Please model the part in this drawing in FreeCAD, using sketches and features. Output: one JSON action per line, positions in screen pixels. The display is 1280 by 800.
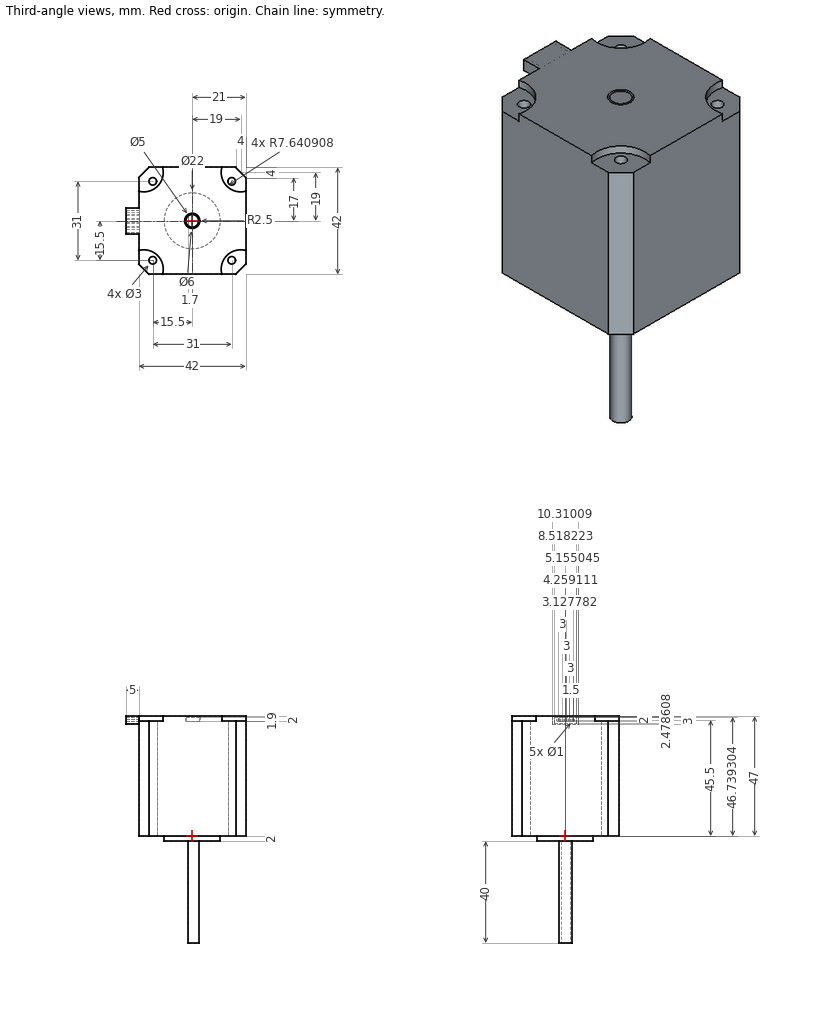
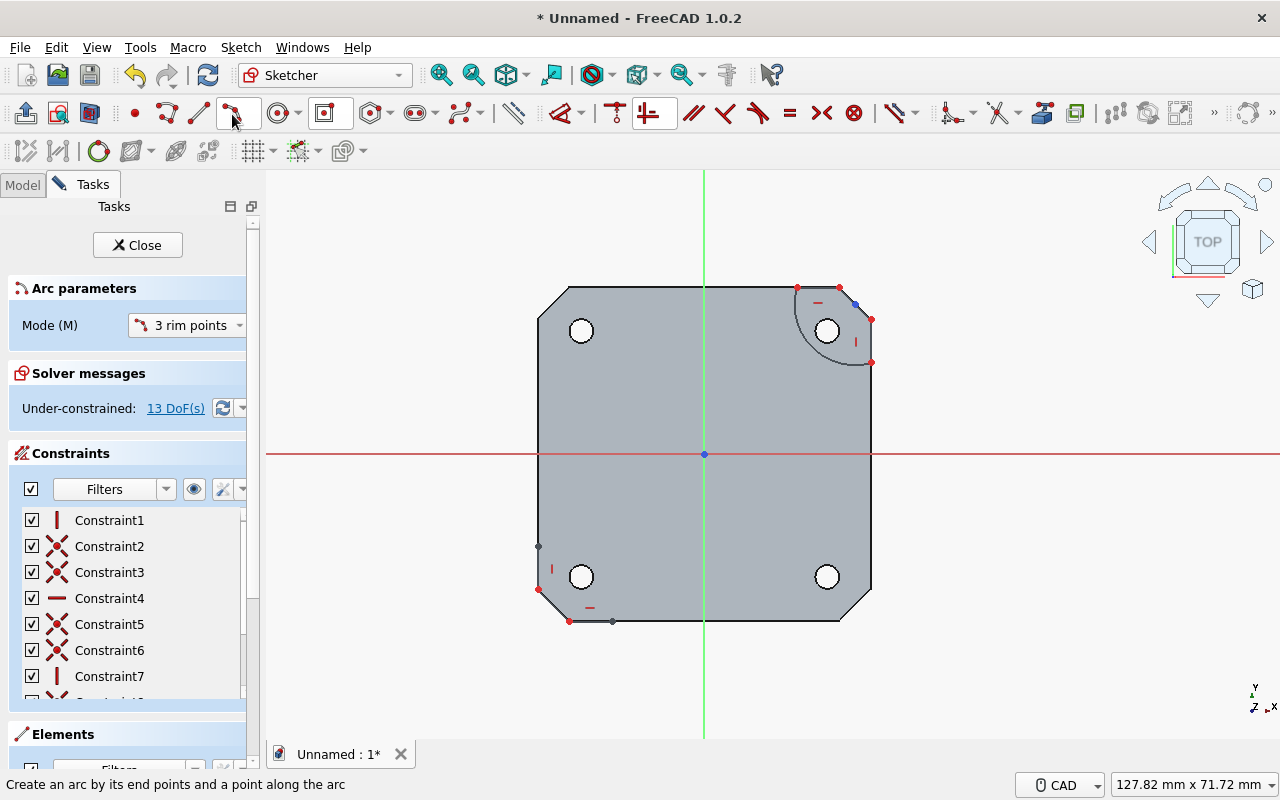
{"action": "left_click", "coordinate": [612, 622]}
{"action": "left_click", "coordinate": [538, 547]}
{"action": "left_click", "coordinate": [596, 562]}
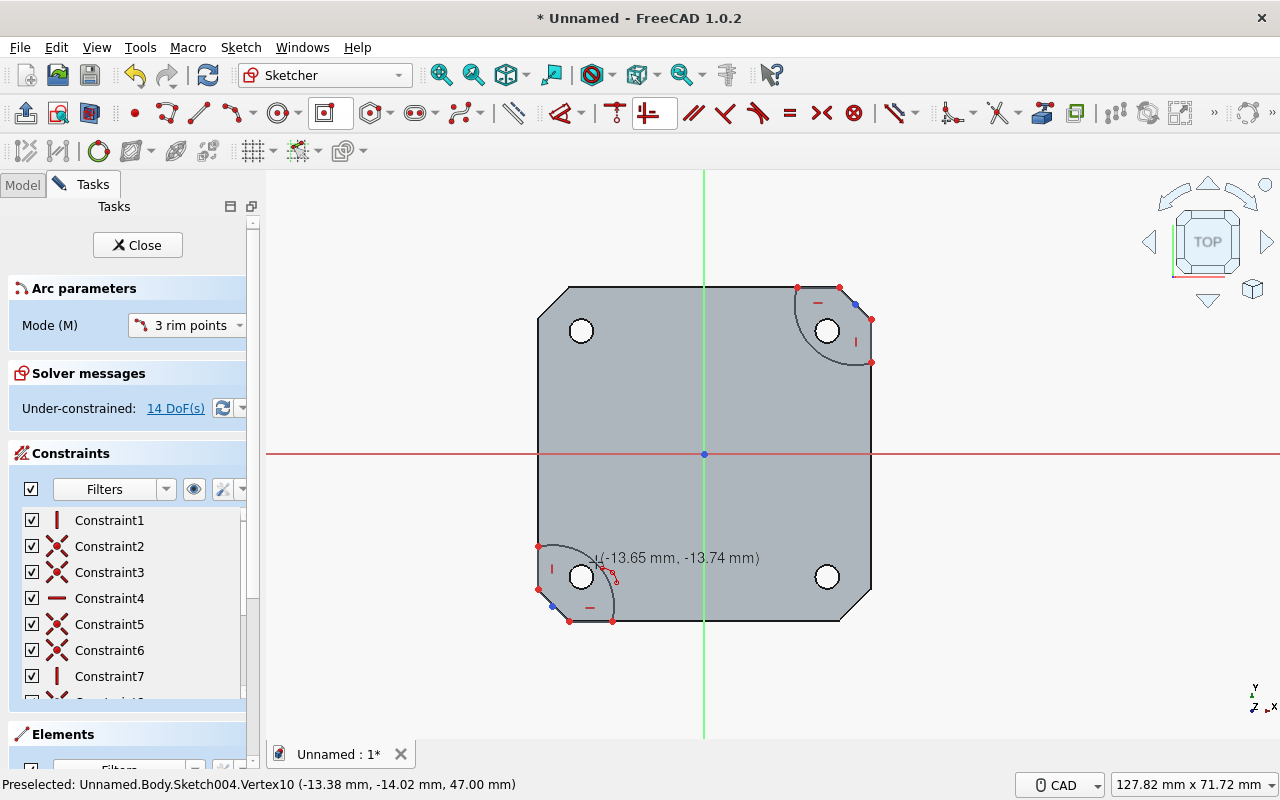
{"action": "key", "text": "g m"}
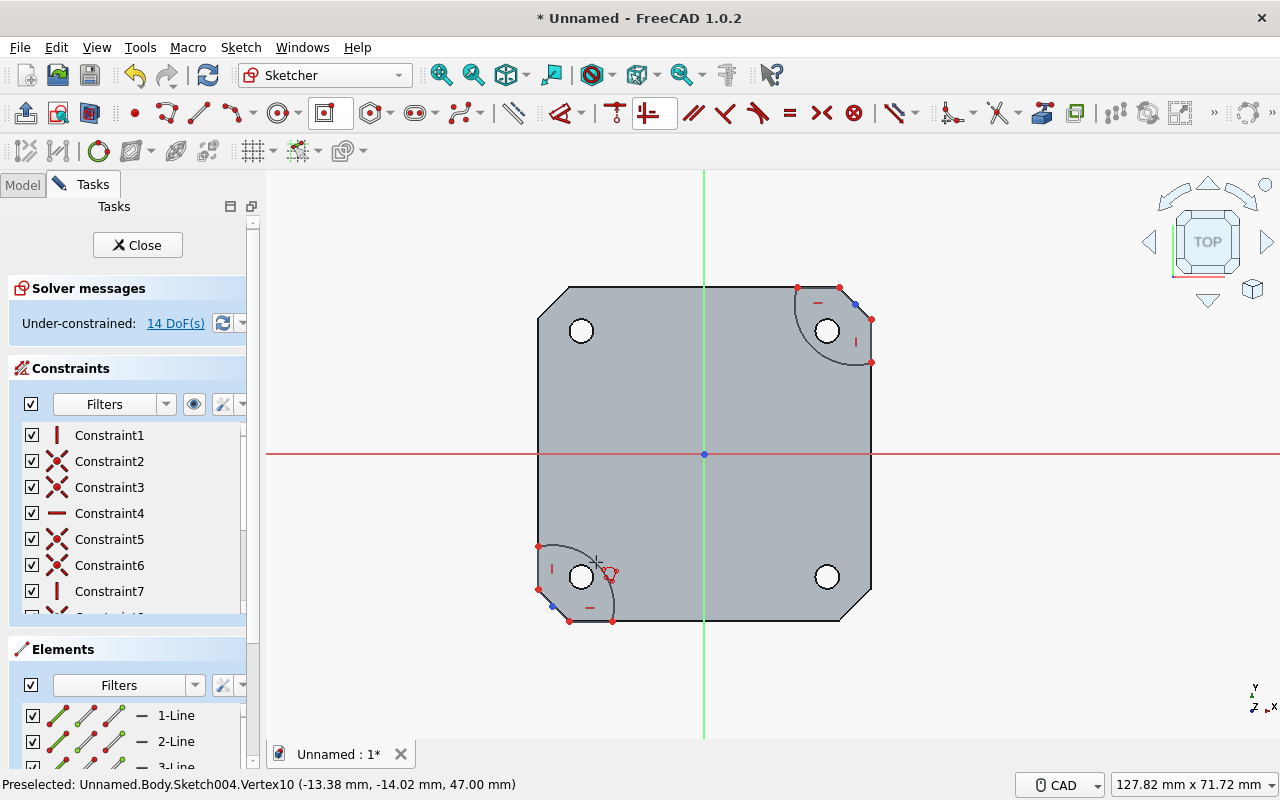
{"action": "left_click", "coordinate": [612, 287]}
{"action": "left_click", "coordinate": [569, 287]}
{"action": "left_click", "coordinate": [538, 319]}
{"action": "left_click", "coordinate": [538, 362]}
{"action": "right_click", "coordinate": [538, 362]}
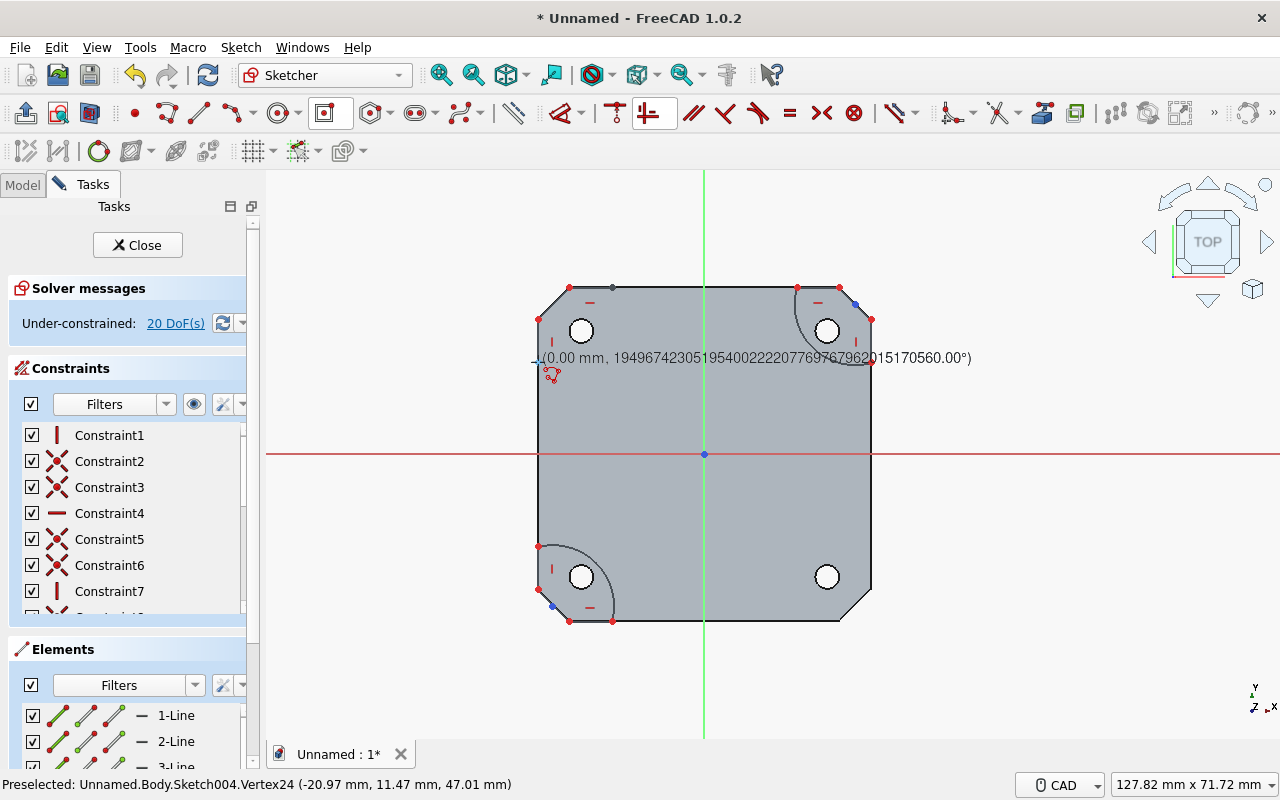
{"action": "left_click", "coordinate": [232, 114]}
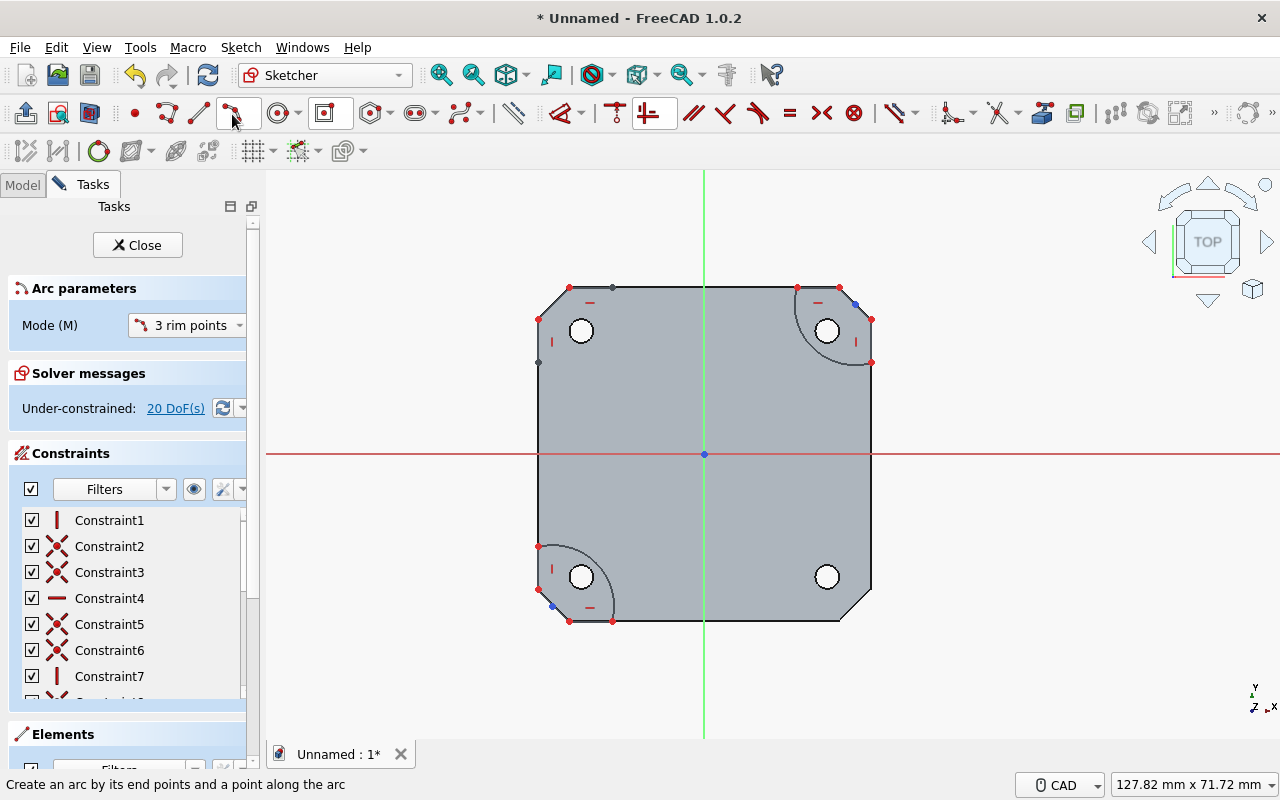
{"action": "left_click", "coordinate": [538, 363]}
{"action": "left_click", "coordinate": [612, 288]}
{"action": "left_click", "coordinate": [596, 346]}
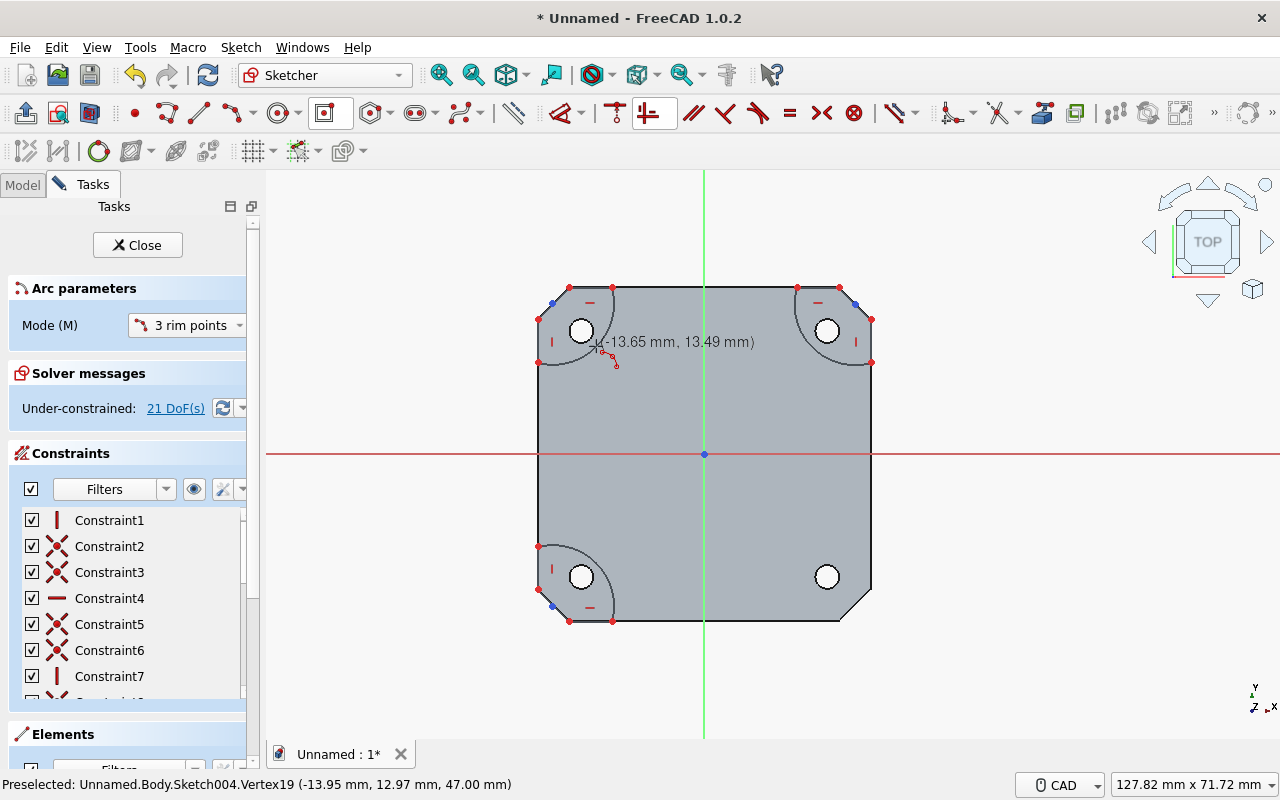
{"action": "left_click", "coordinate": [168, 114]}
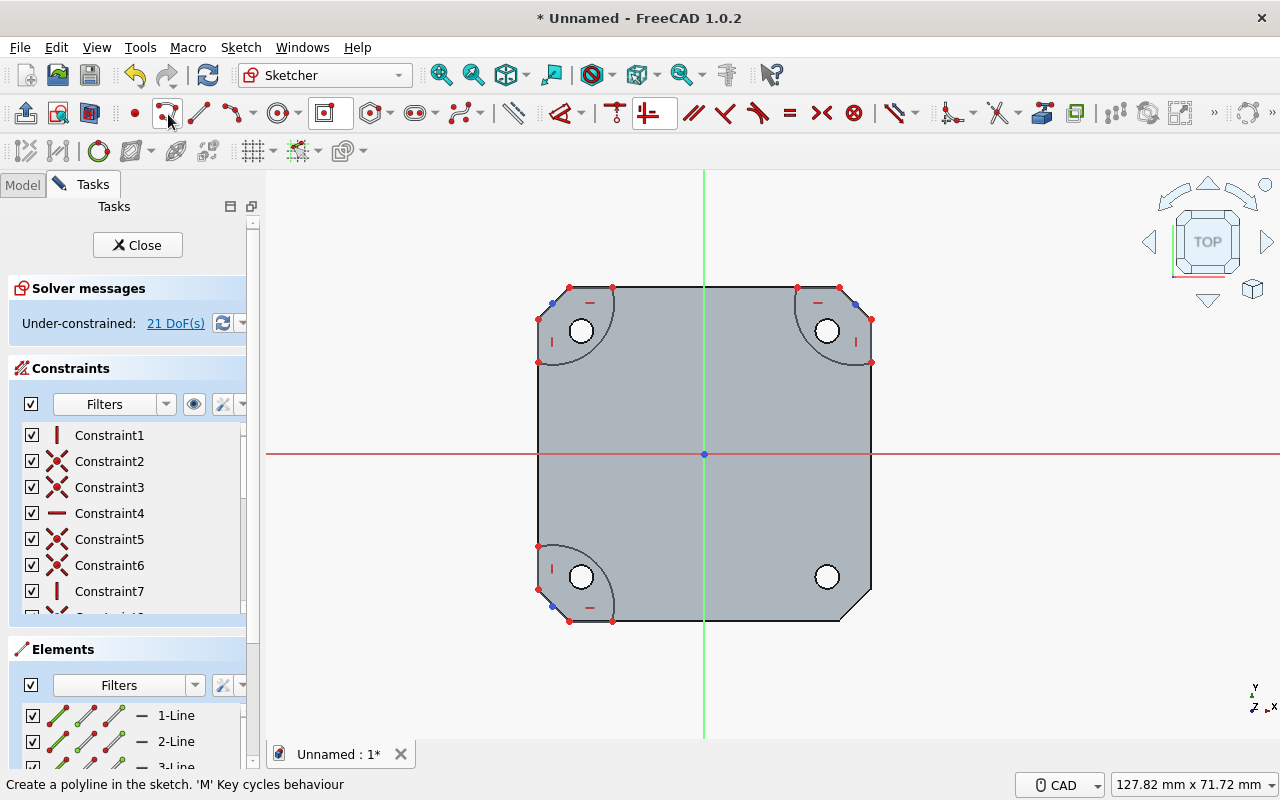
{"action": "left_click", "coordinate": [797, 621]}
{"action": "left_click", "coordinate": [839, 621]}
{"action": "left_click", "coordinate": [871, 589]}
{"action": "left_click", "coordinate": [871, 546]}
{"action": "right_click", "coordinate": [871, 546]}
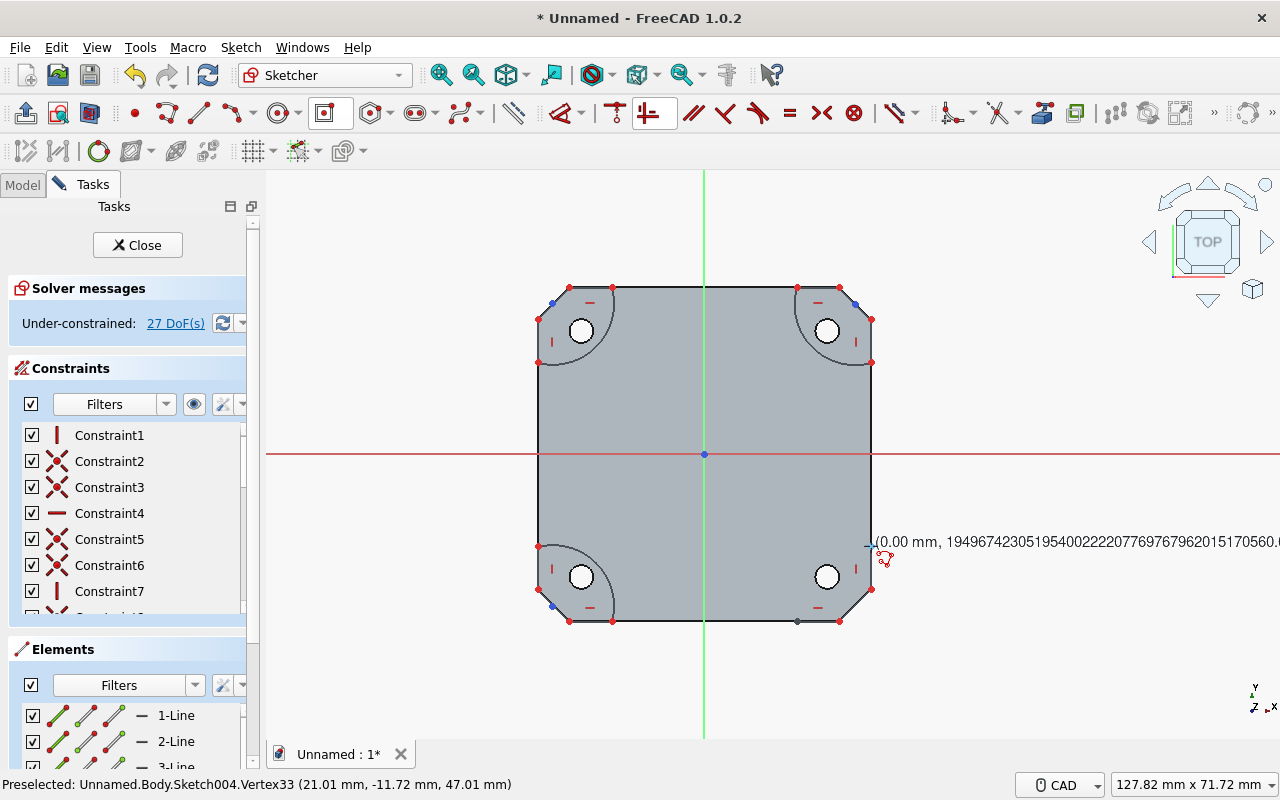
{"action": "key", "text": "g 3 a"}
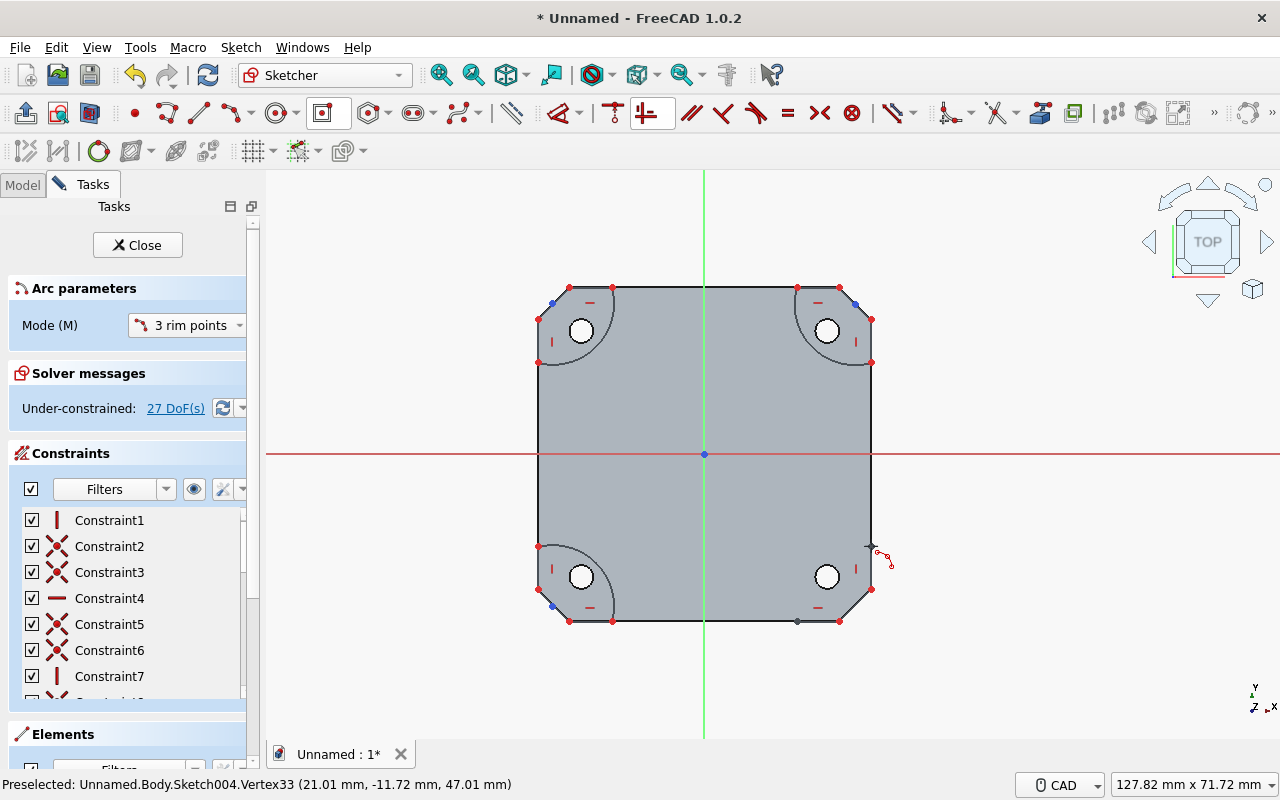
{"action": "left_click", "coordinate": [871, 547]}
{"action": "left_click", "coordinate": [797, 622]}
{"action": "left_click", "coordinate": [812, 562]}
{"action": "key", "text": "Escape"}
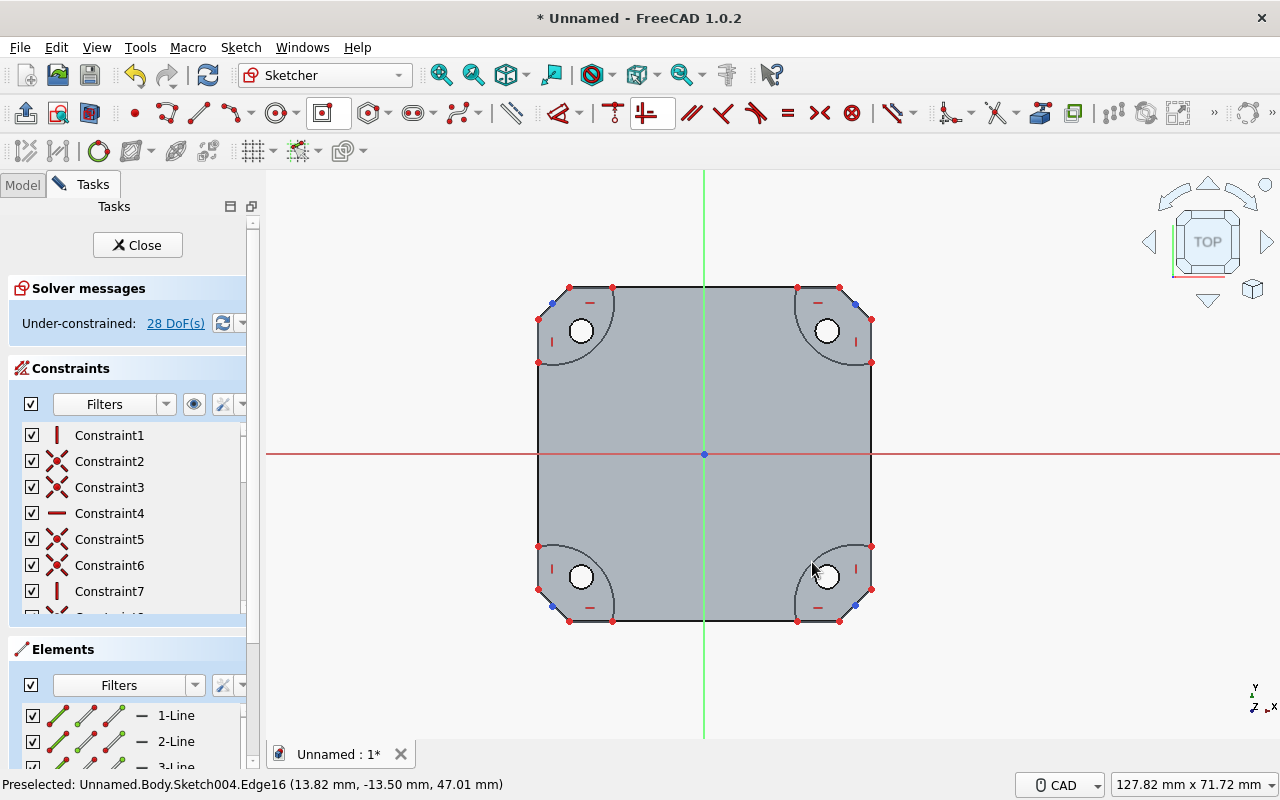
{"action": "left_click", "coordinate": [798, 326]}